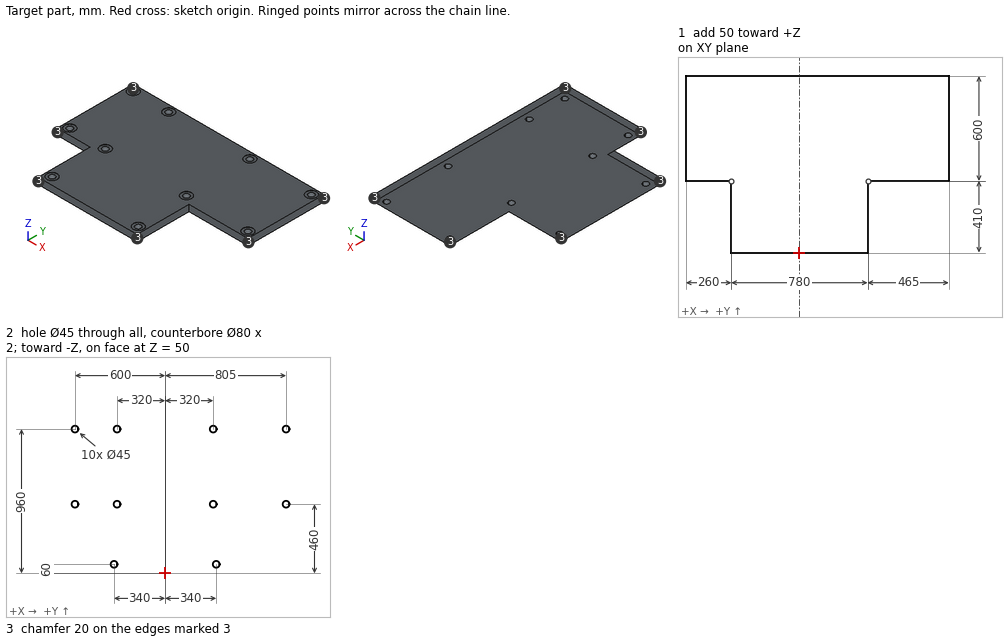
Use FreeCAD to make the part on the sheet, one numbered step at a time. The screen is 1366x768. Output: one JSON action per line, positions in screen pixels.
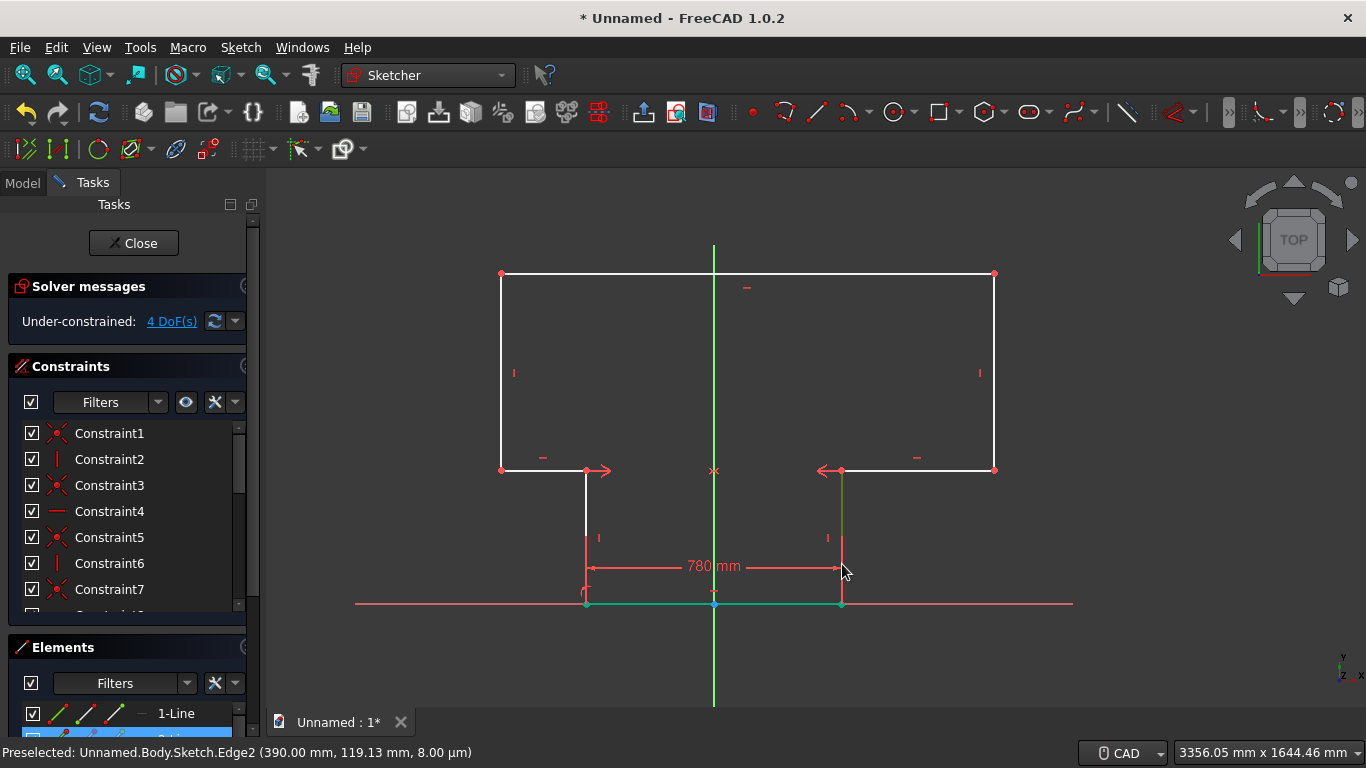
{"action": "left_click", "coordinate": [1196, 112]}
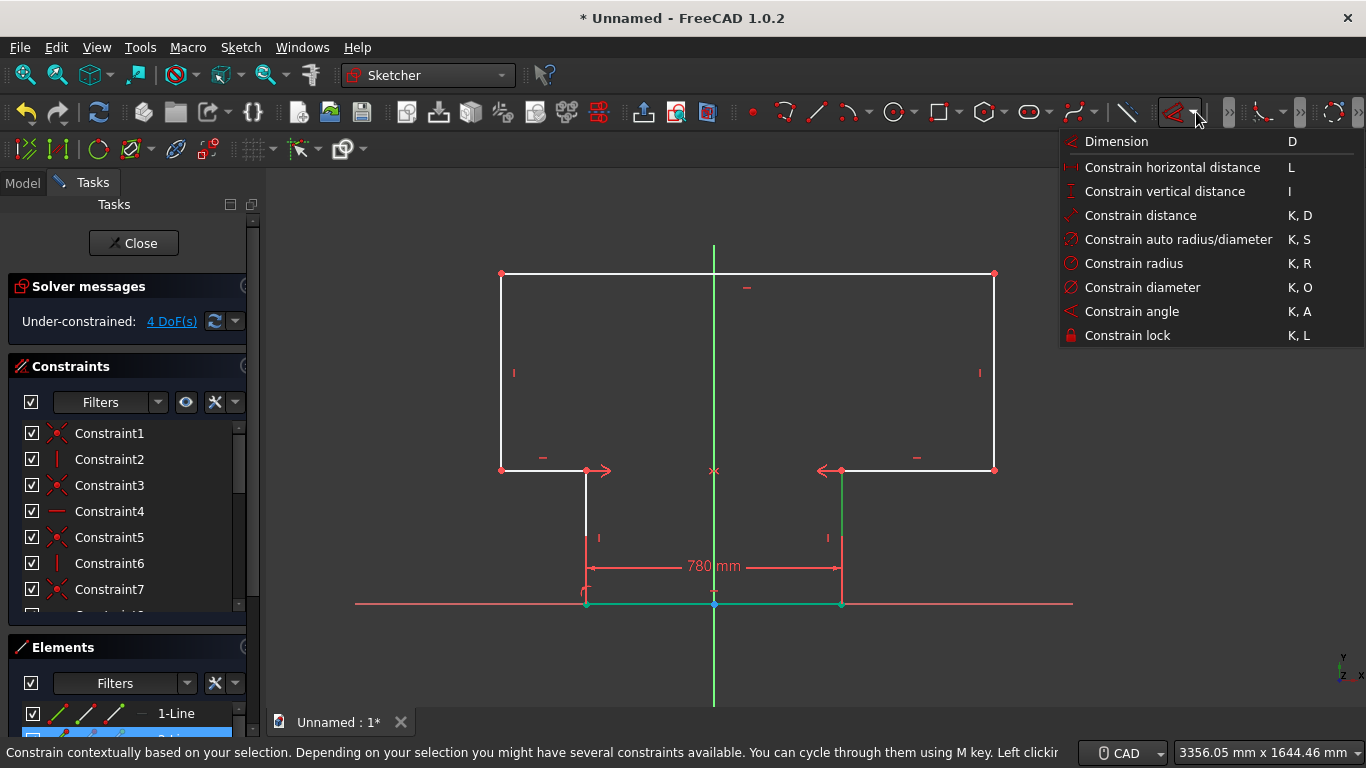
{"action": "left_click", "coordinate": [1212, 191]}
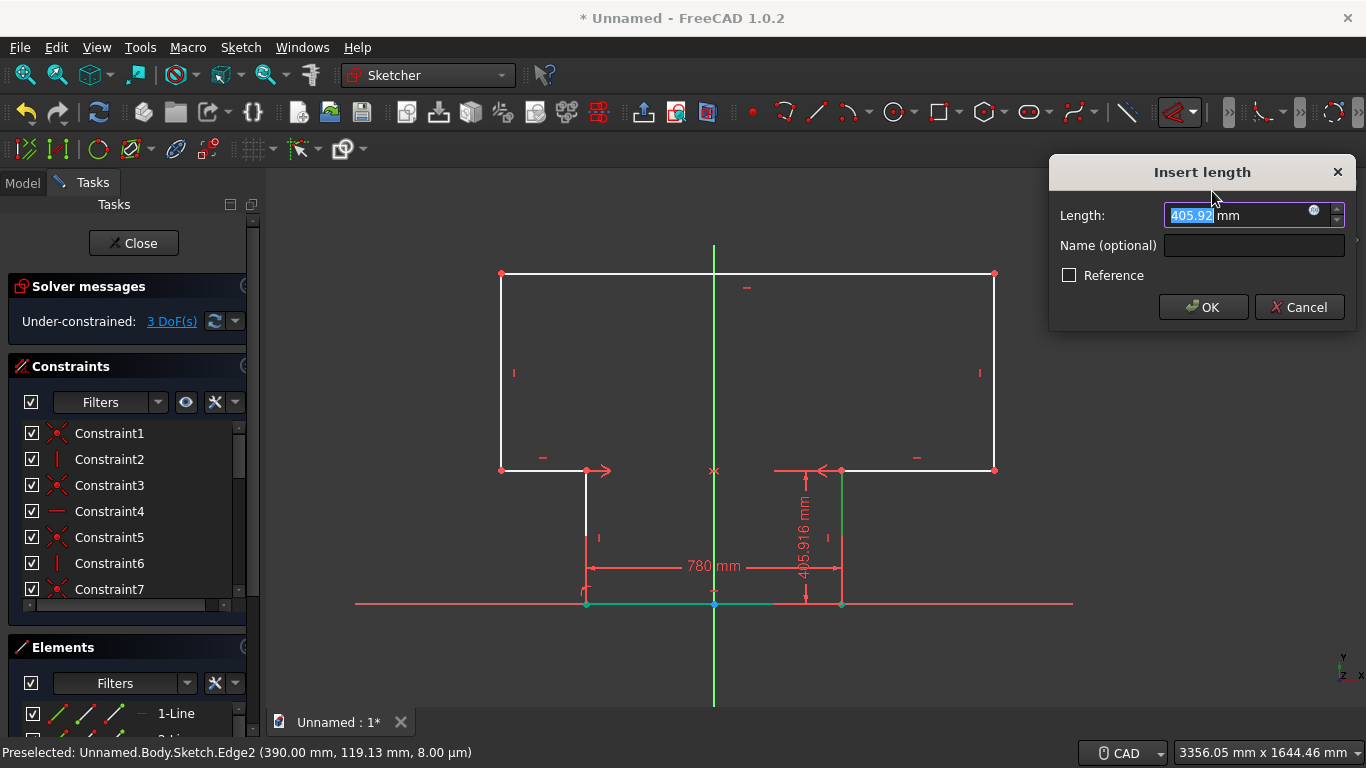
{"action": "type", "text": "410"}
{"action": "key", "text": "Return"}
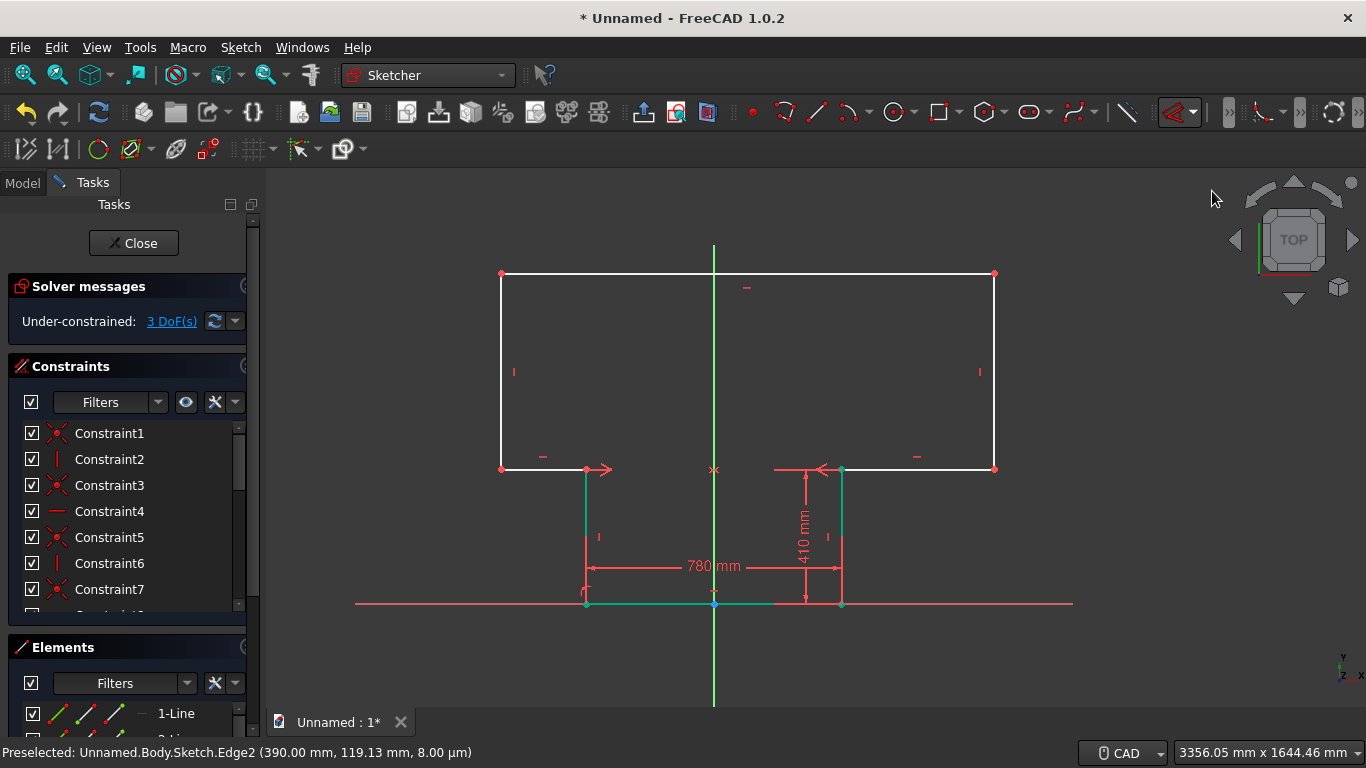
{"action": "left_click", "coordinate": [887, 470]}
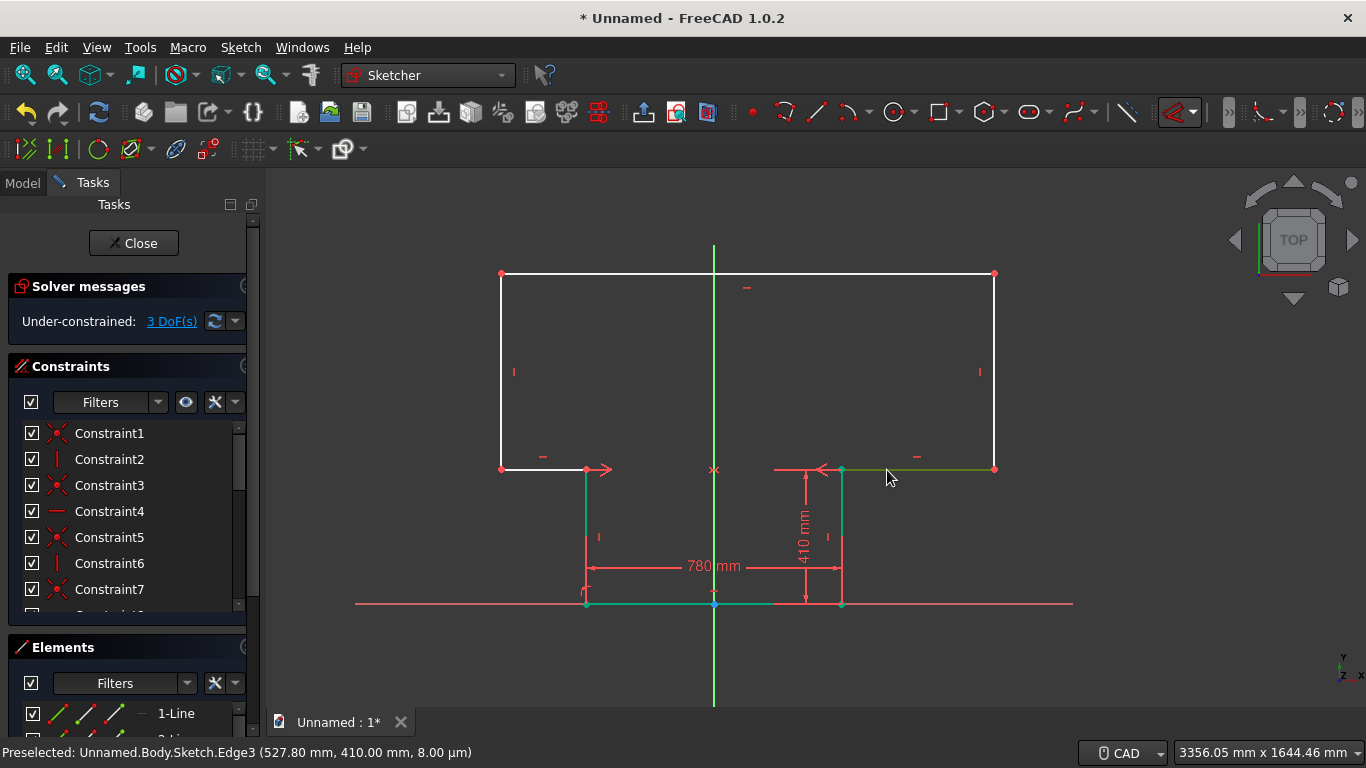
{"action": "key", "text": "l"}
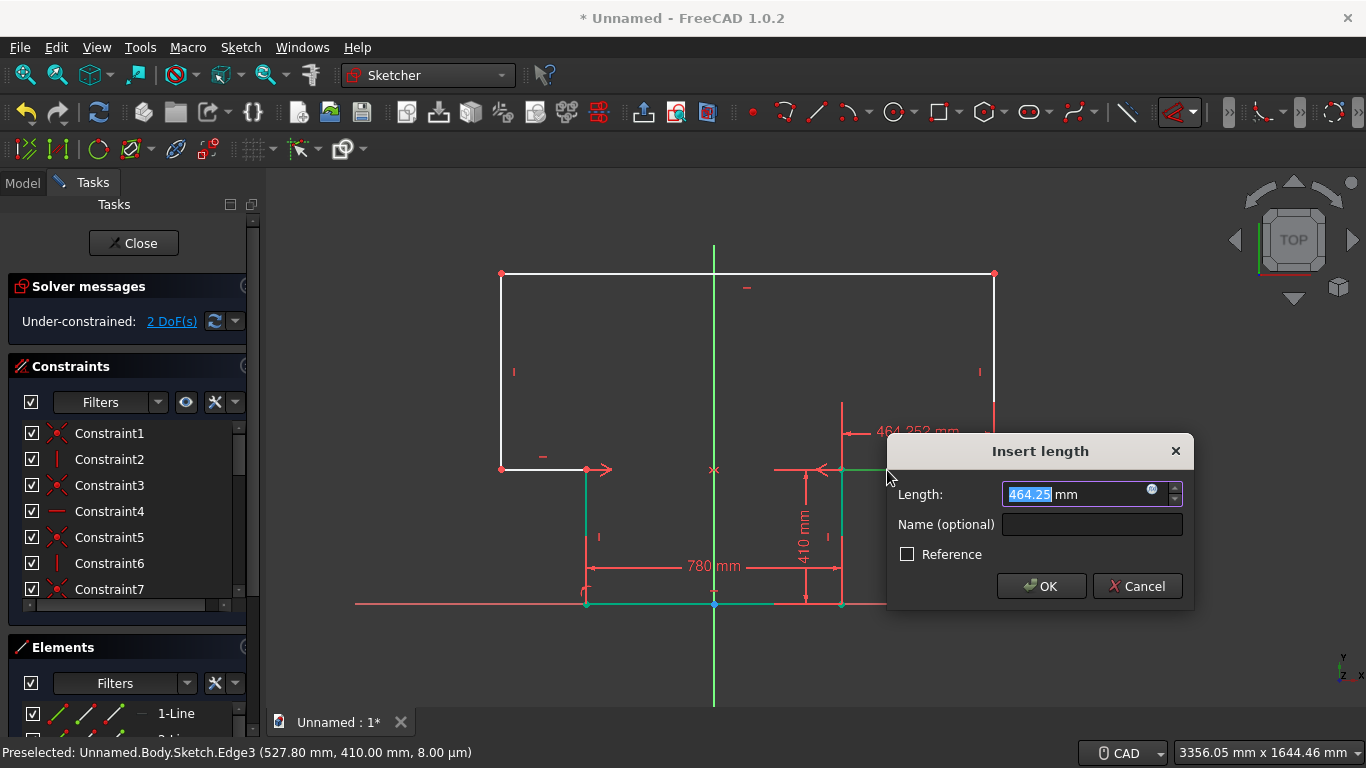
{"action": "type", "text": "465"}
{"action": "key", "text": "Return"}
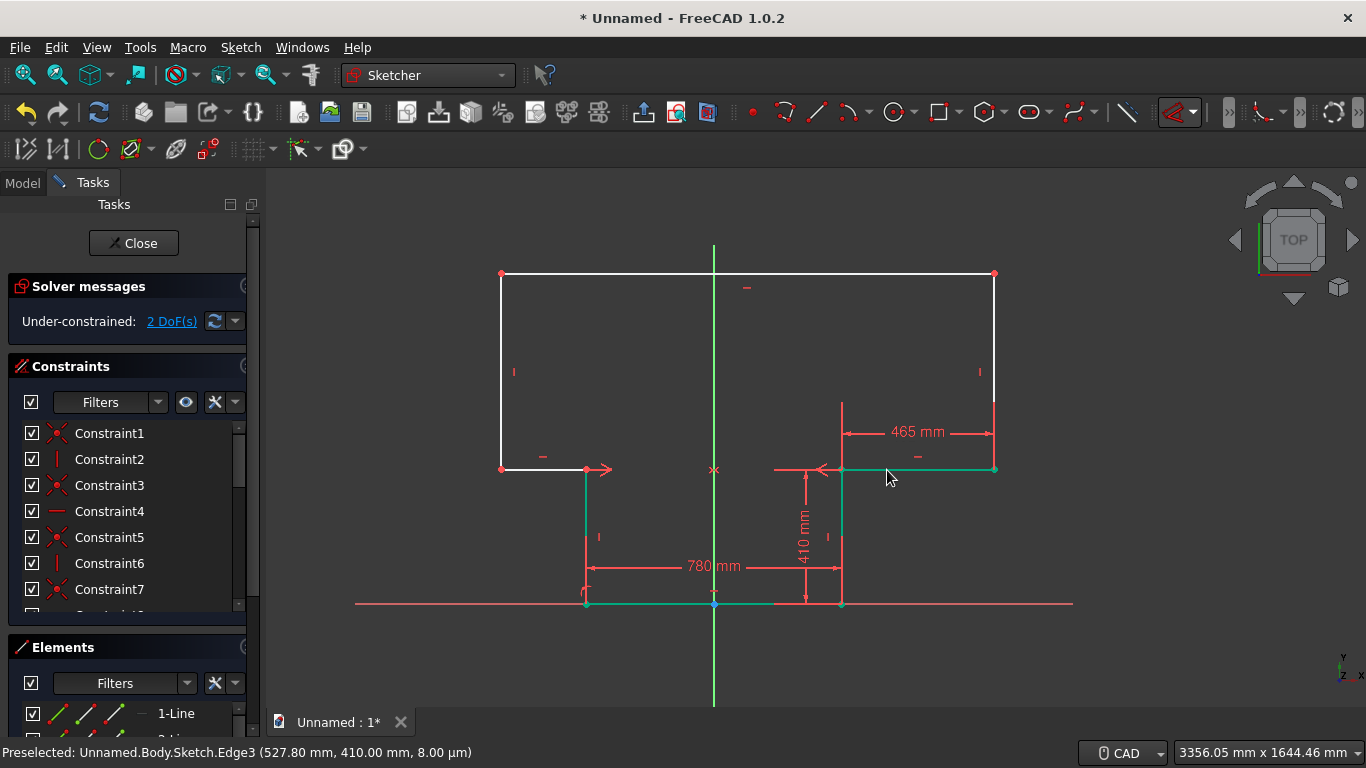
{"action": "left_click", "coordinate": [994, 411]}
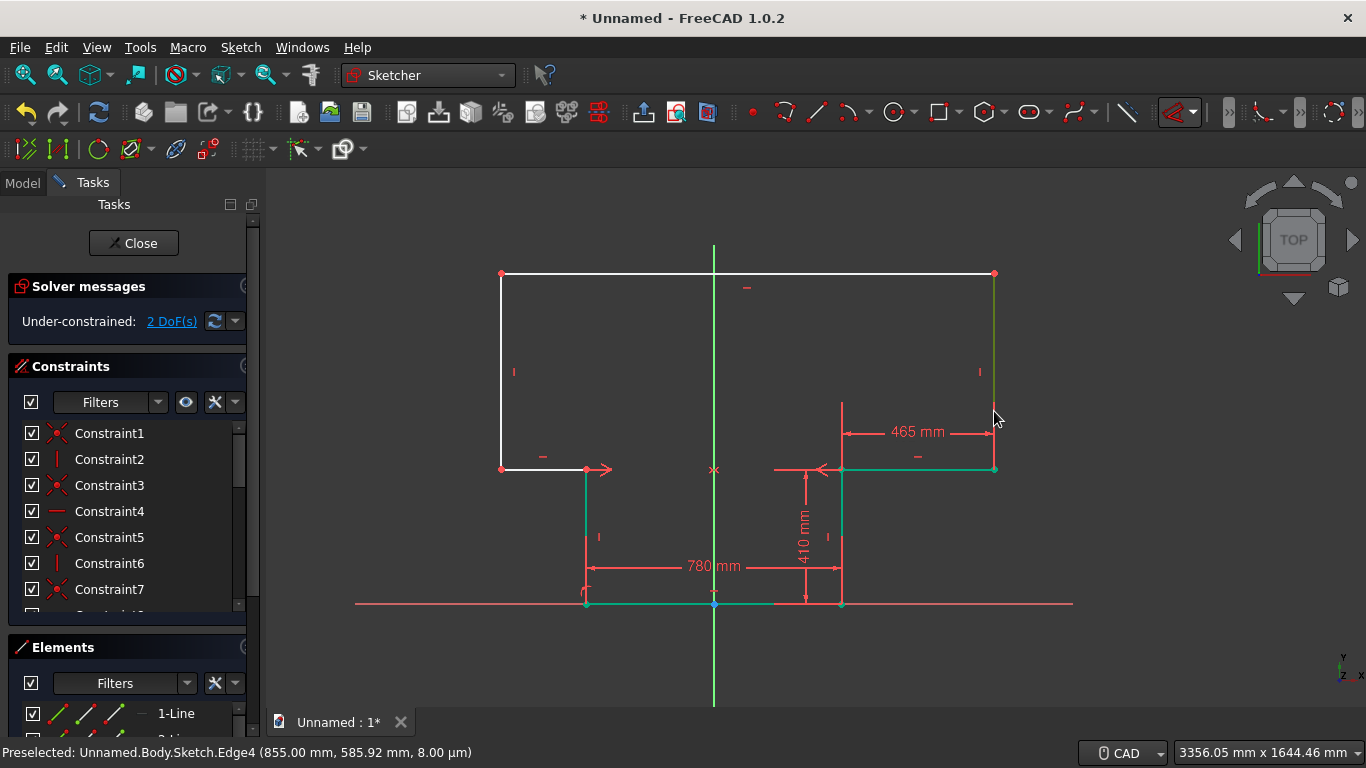
{"action": "key", "text": "i"}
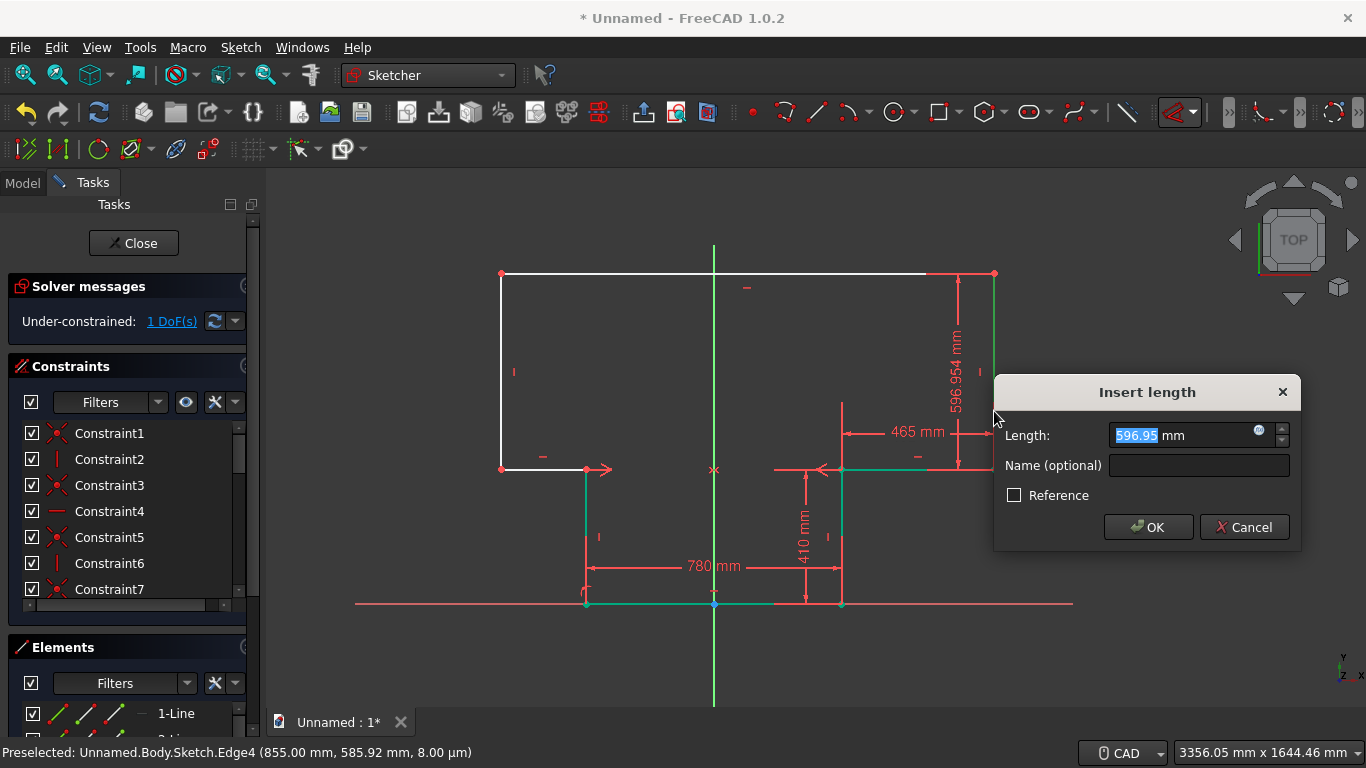
{"action": "type", "text": "600"}
{"action": "key", "text": "Return"}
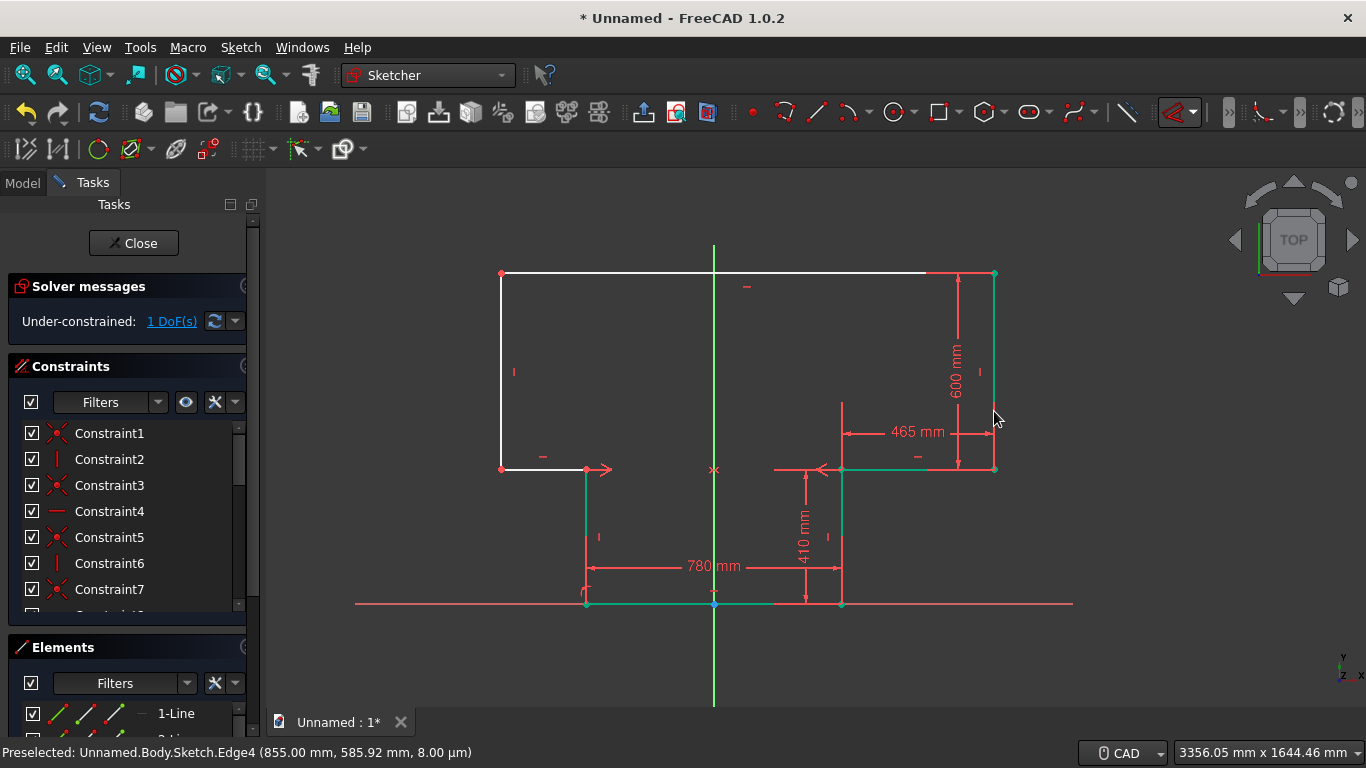
{"action": "left_click", "coordinate": [527, 470]}